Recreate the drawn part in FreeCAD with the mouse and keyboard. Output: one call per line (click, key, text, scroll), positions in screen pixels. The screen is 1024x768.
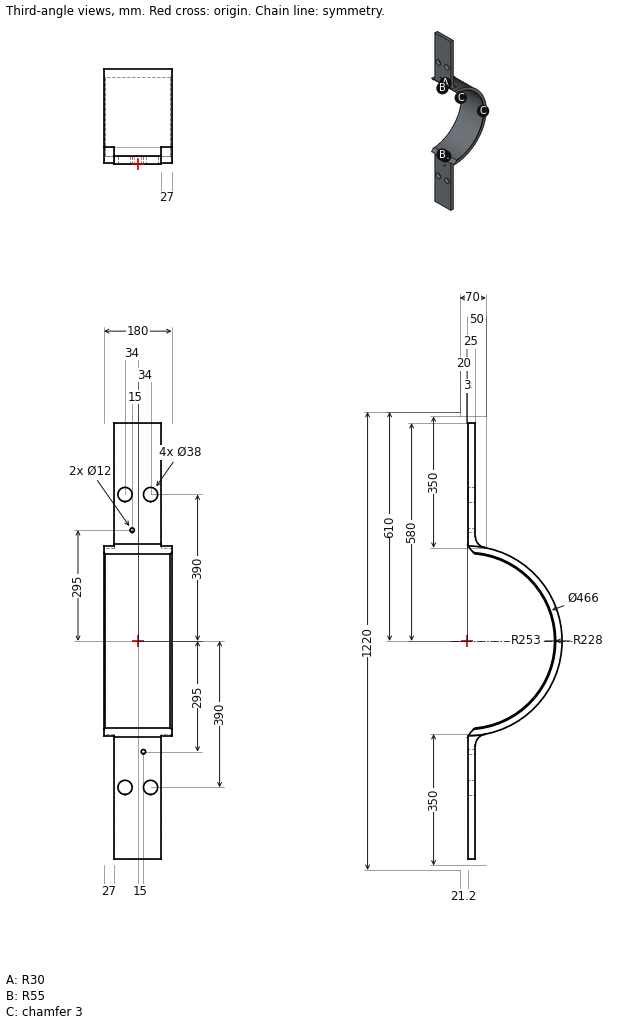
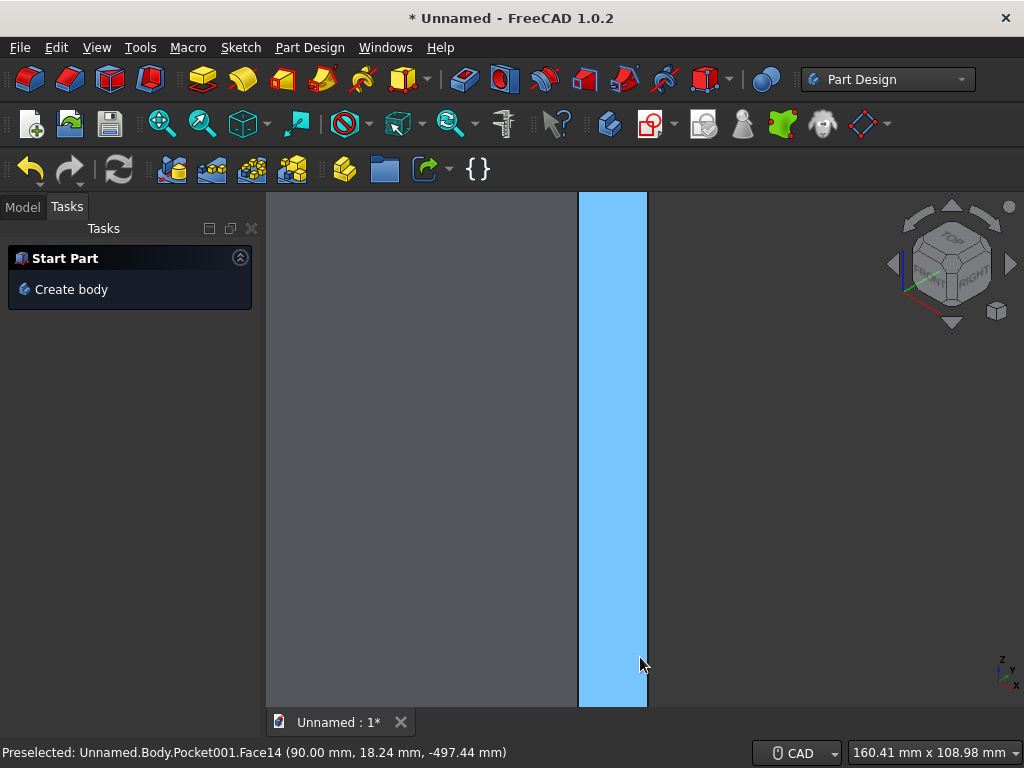
click(638, 655)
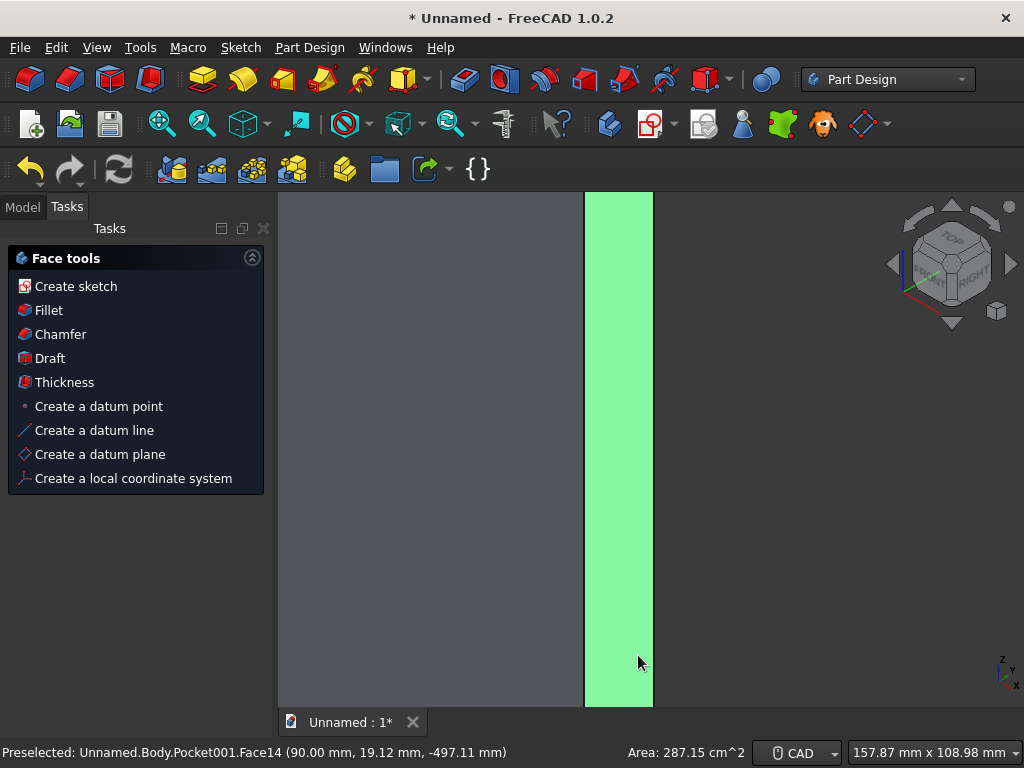
click(650, 124)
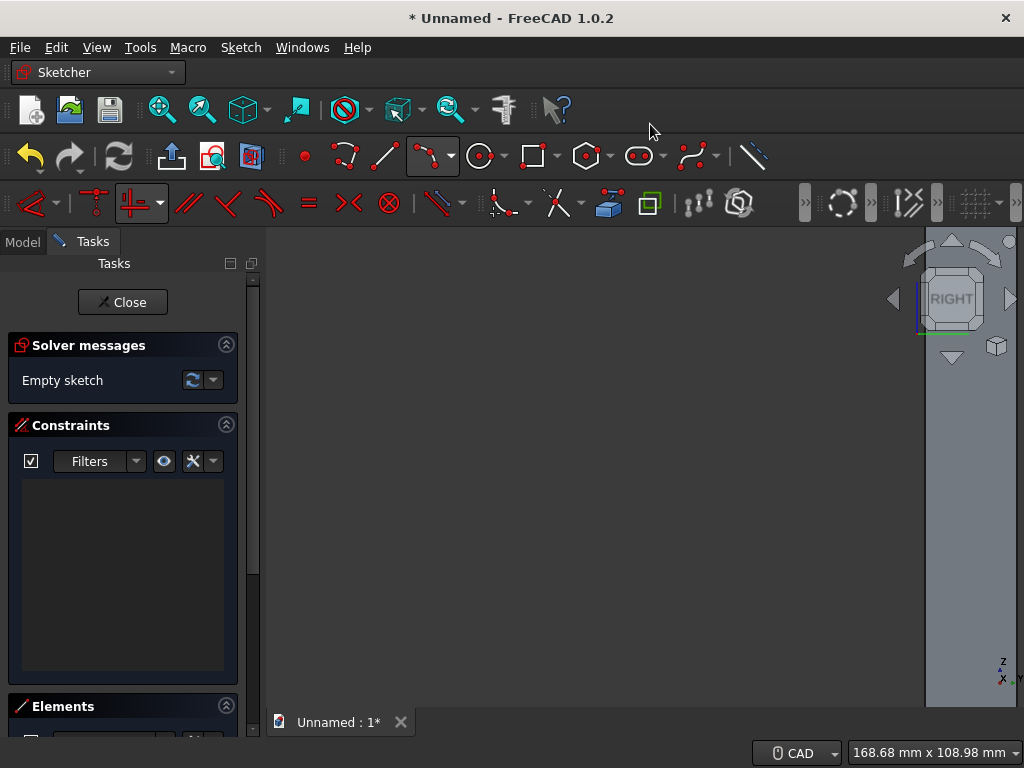
scroll(544, 679, down, 13)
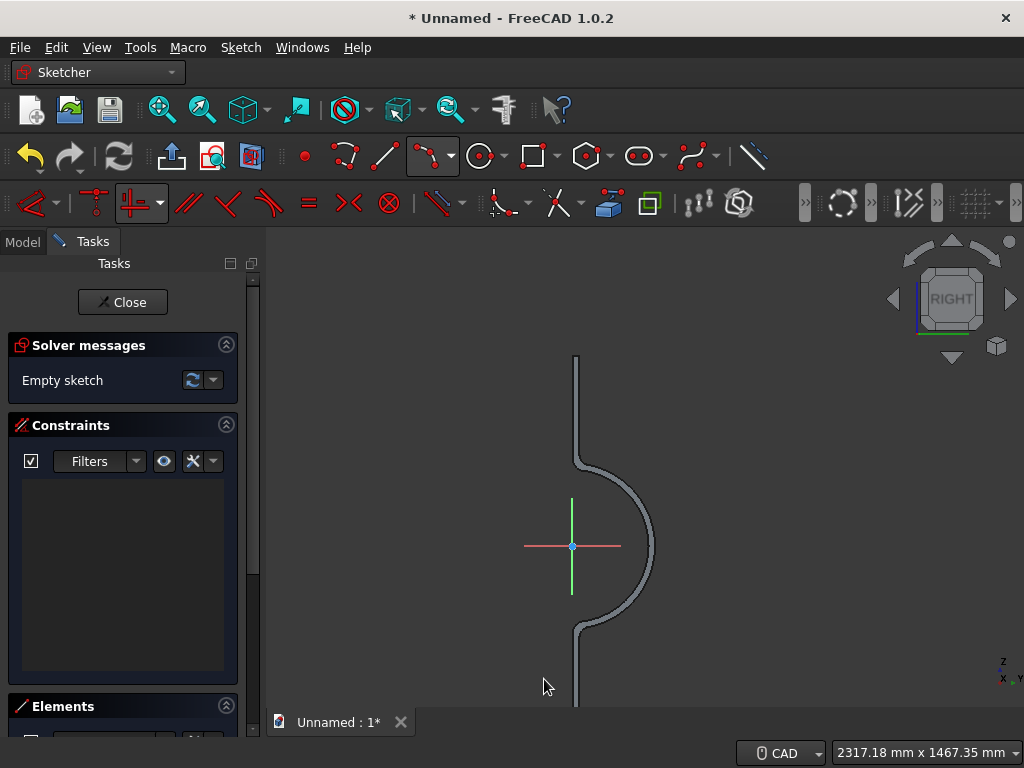
scroll(579, 410, up, 2)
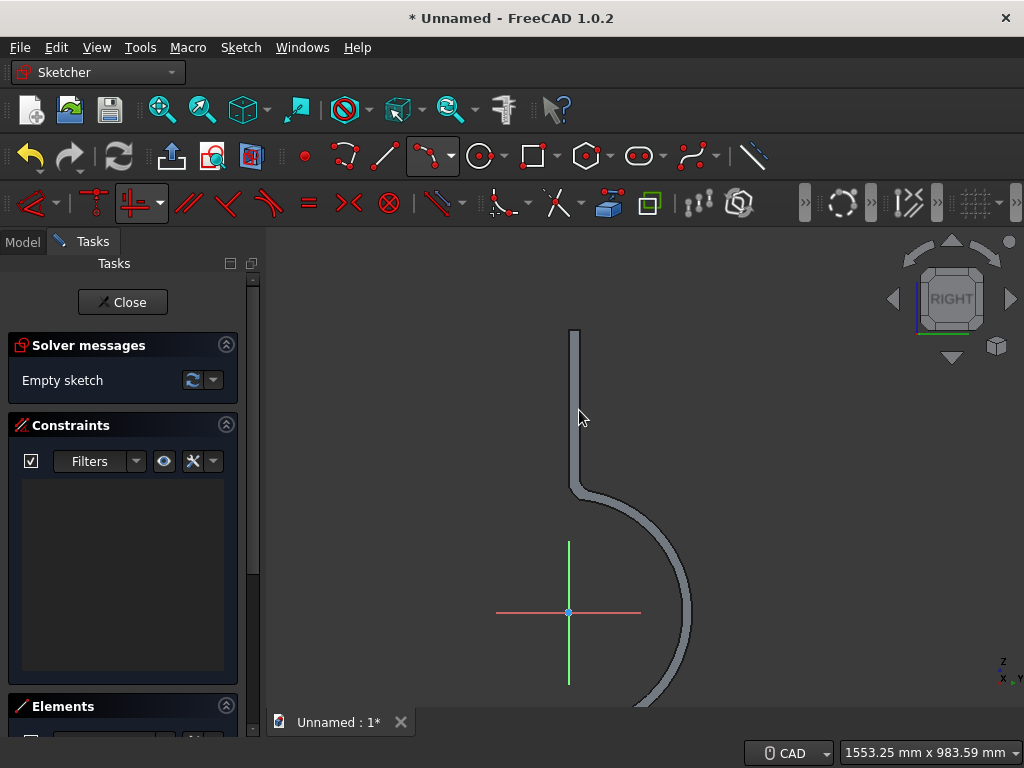
click(346, 156)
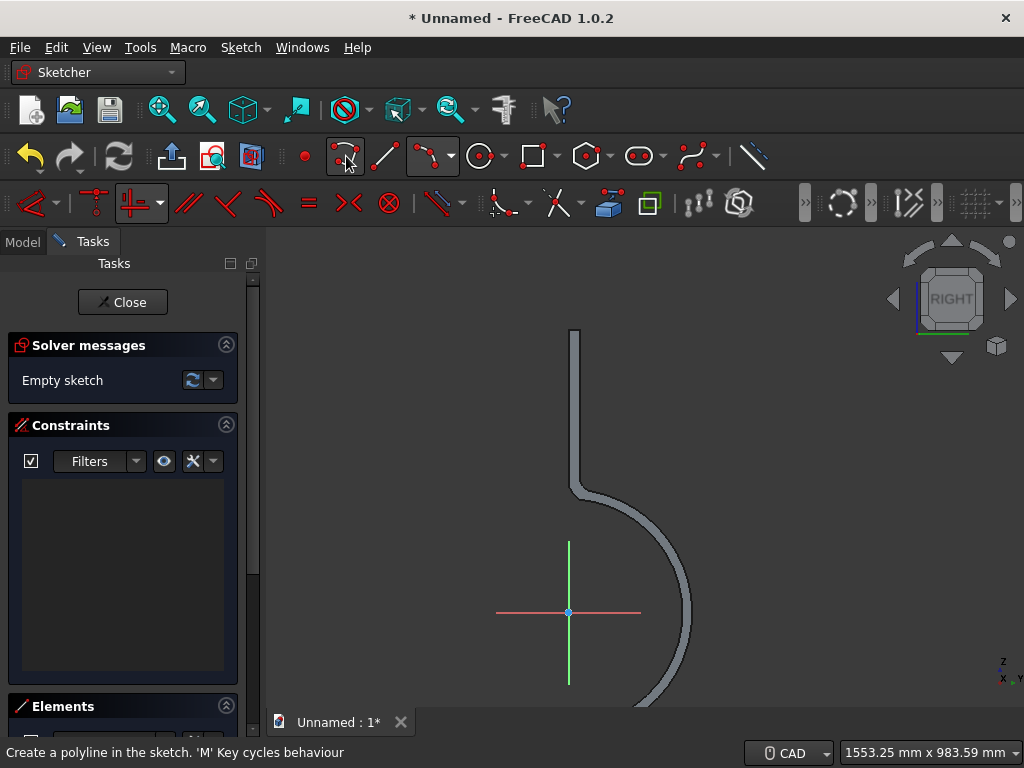
click(593, 492)
click(593, 321)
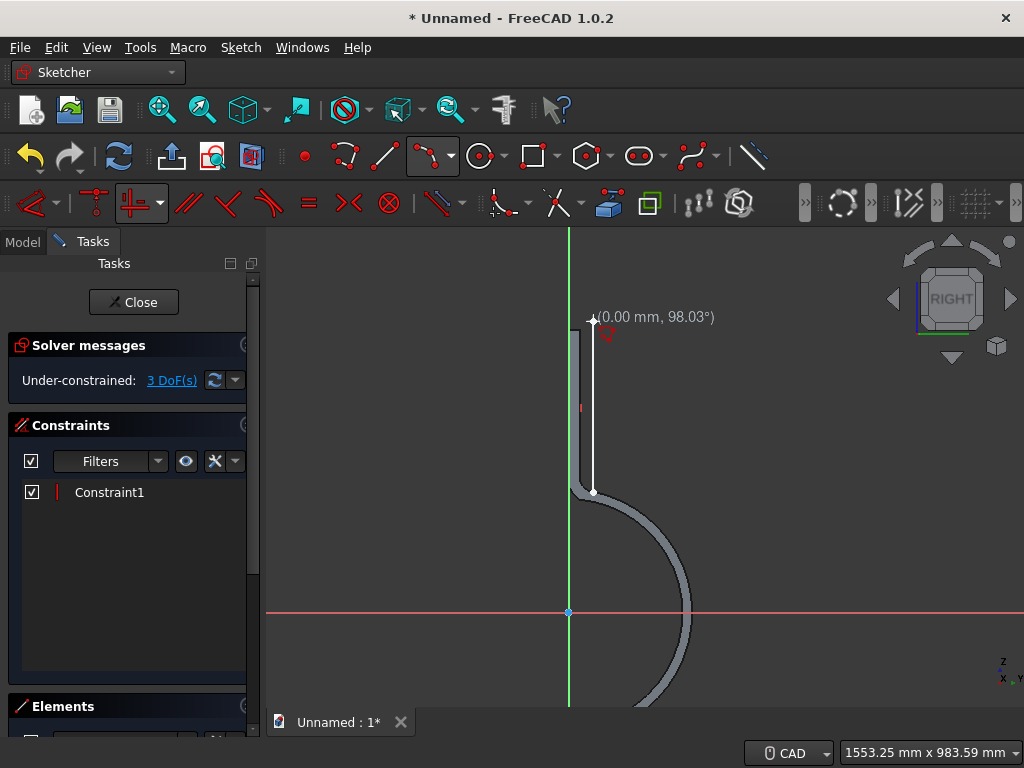
scroll(559, 321, up, 3)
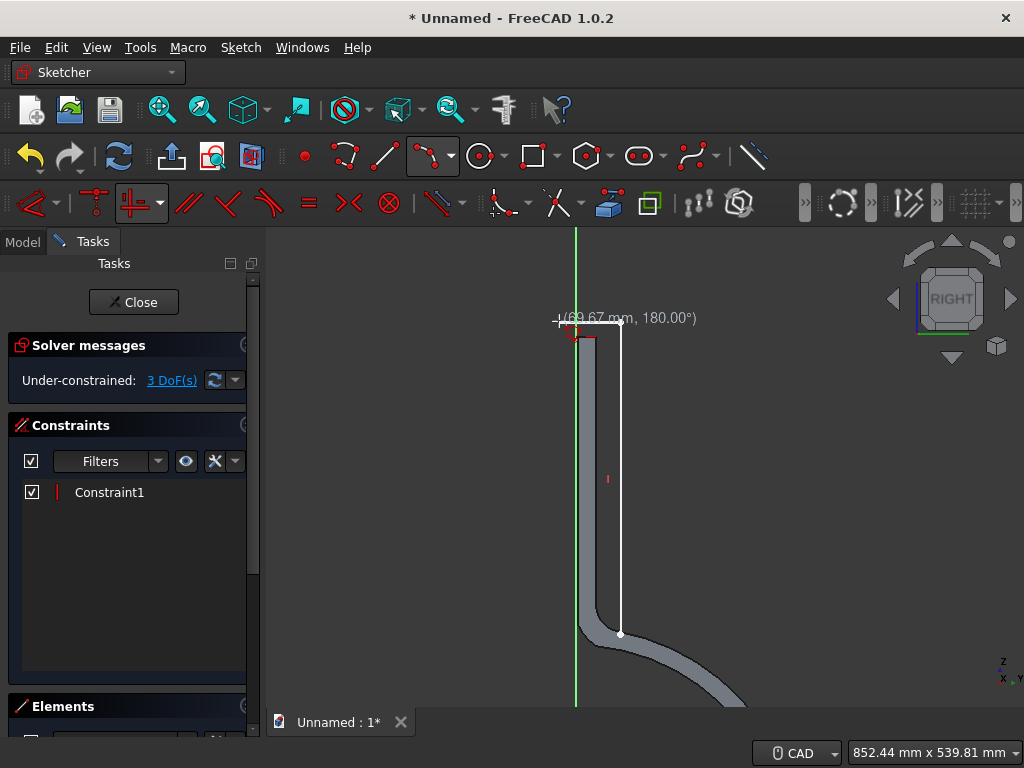
click(559, 321)
click(559, 628)
right_click(559, 628)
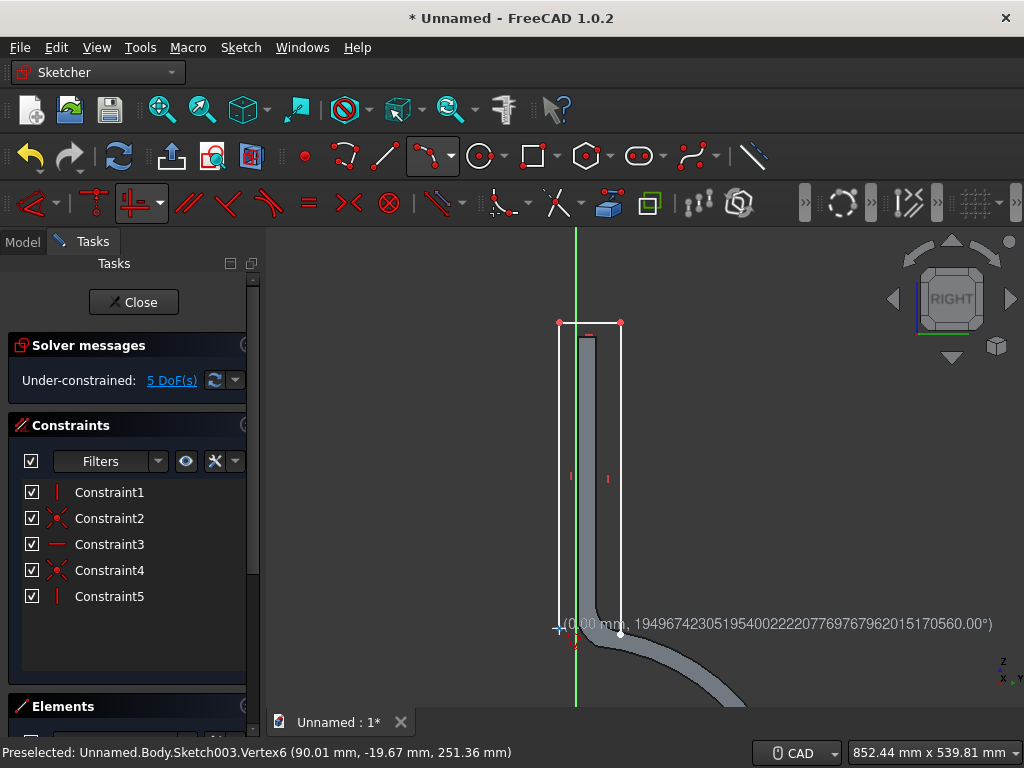
click(426, 156)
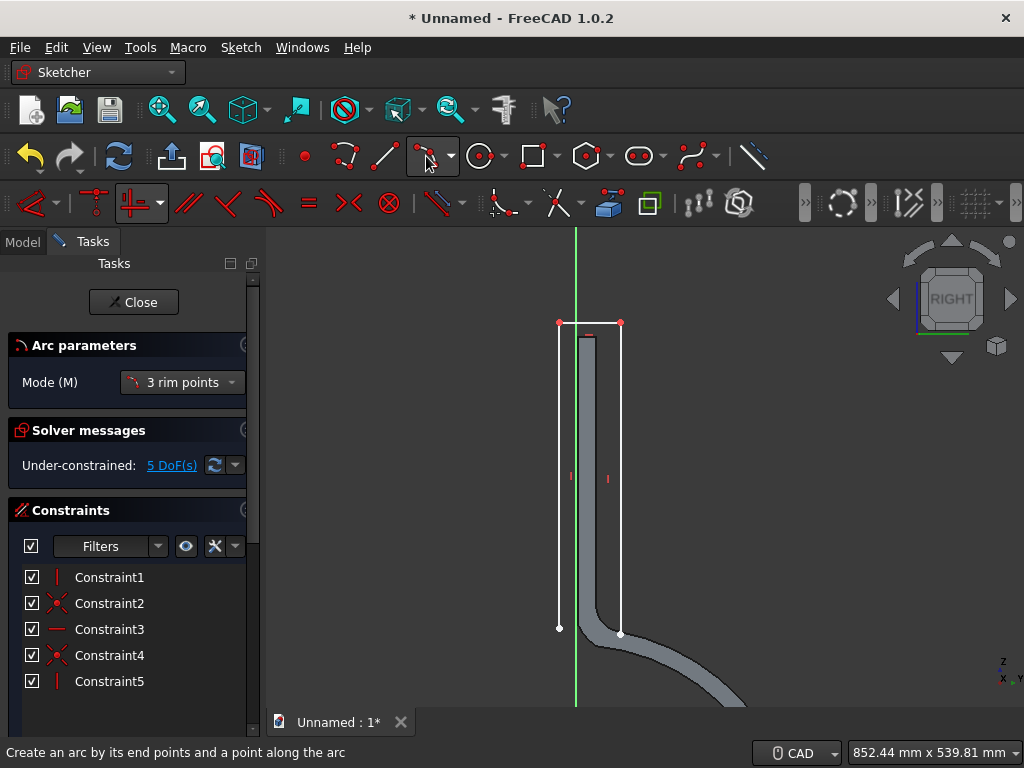
click(559, 629)
click(621, 634)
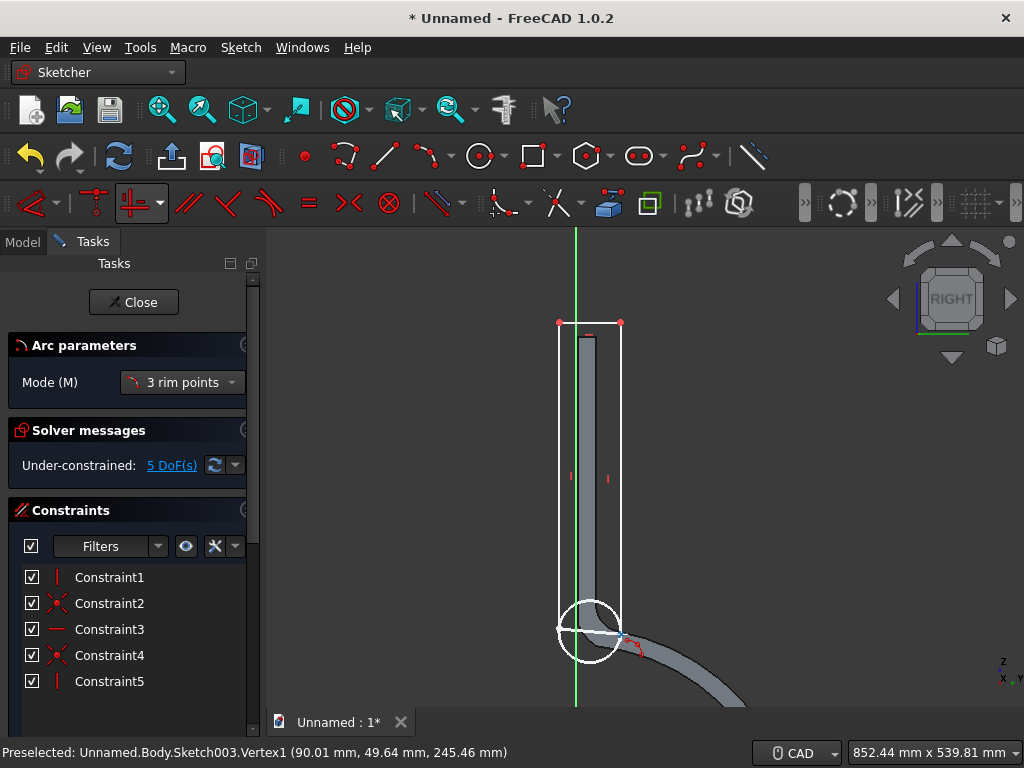
scroll(590, 628, up, 10)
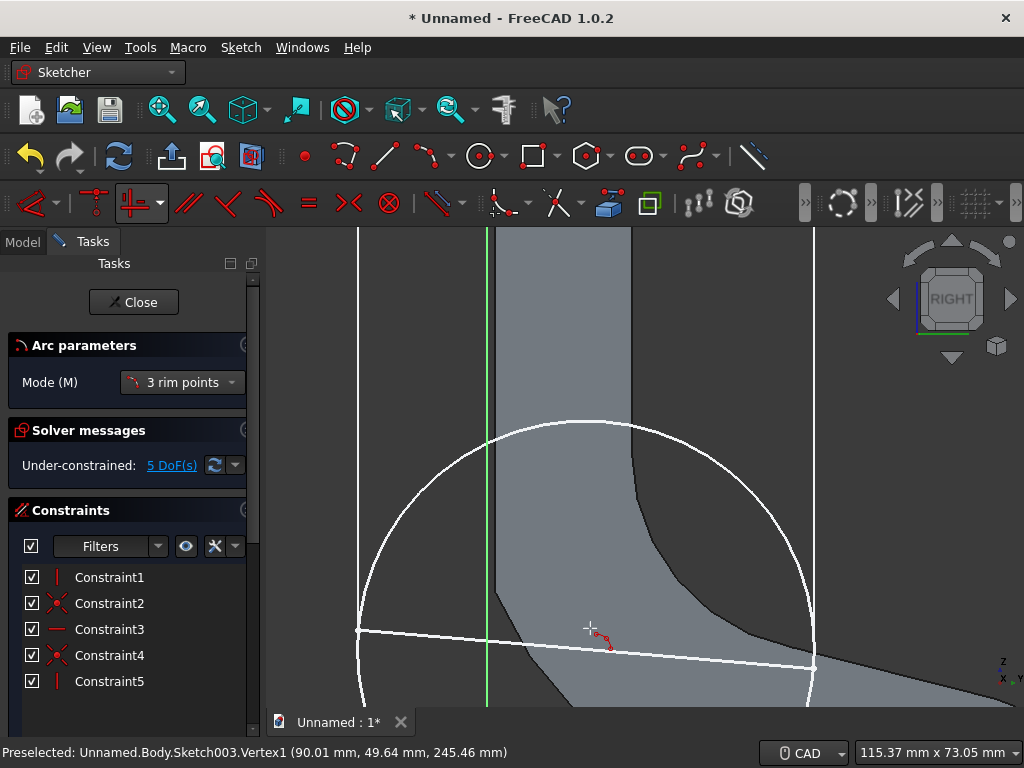
click(587, 622)
key(Escape)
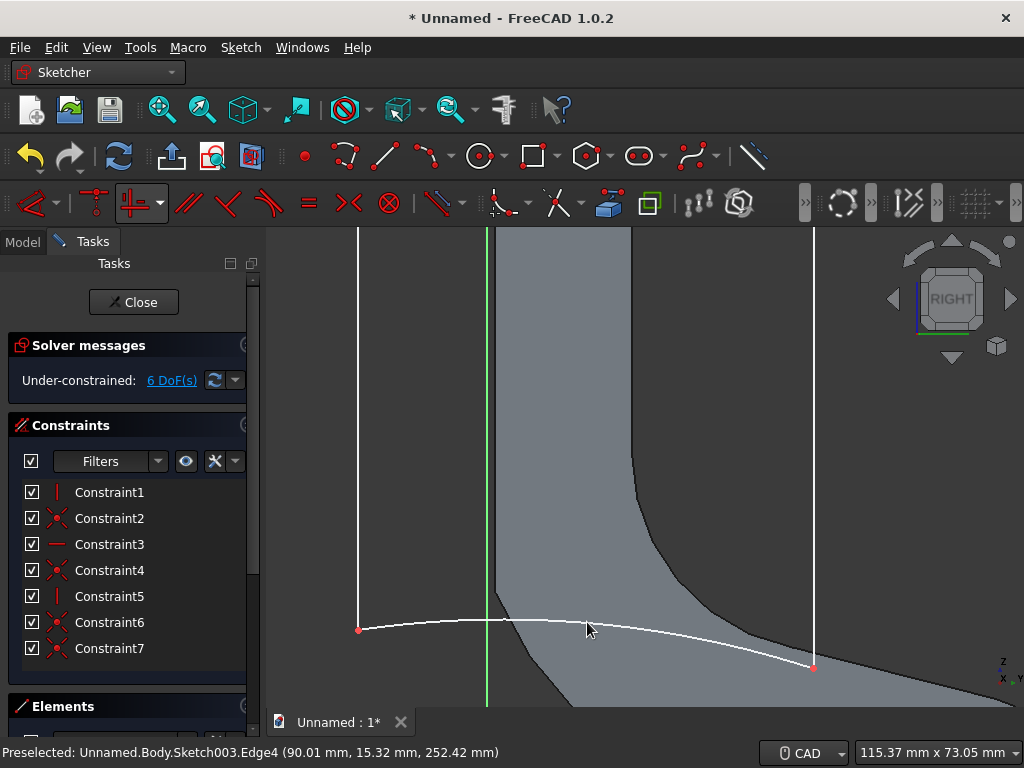
scroll(576, 479, down, 13)